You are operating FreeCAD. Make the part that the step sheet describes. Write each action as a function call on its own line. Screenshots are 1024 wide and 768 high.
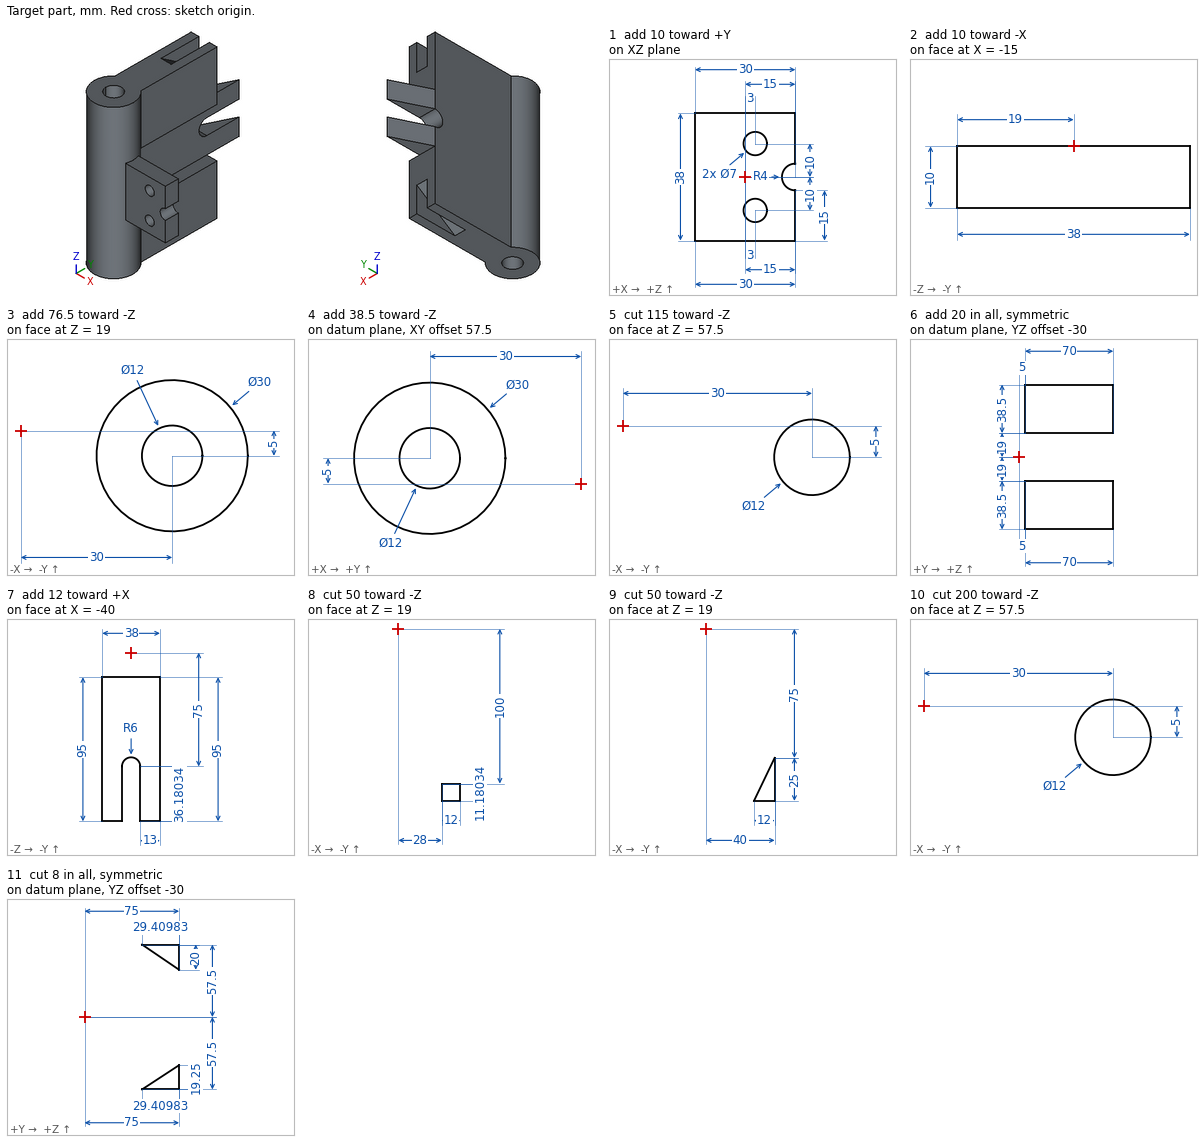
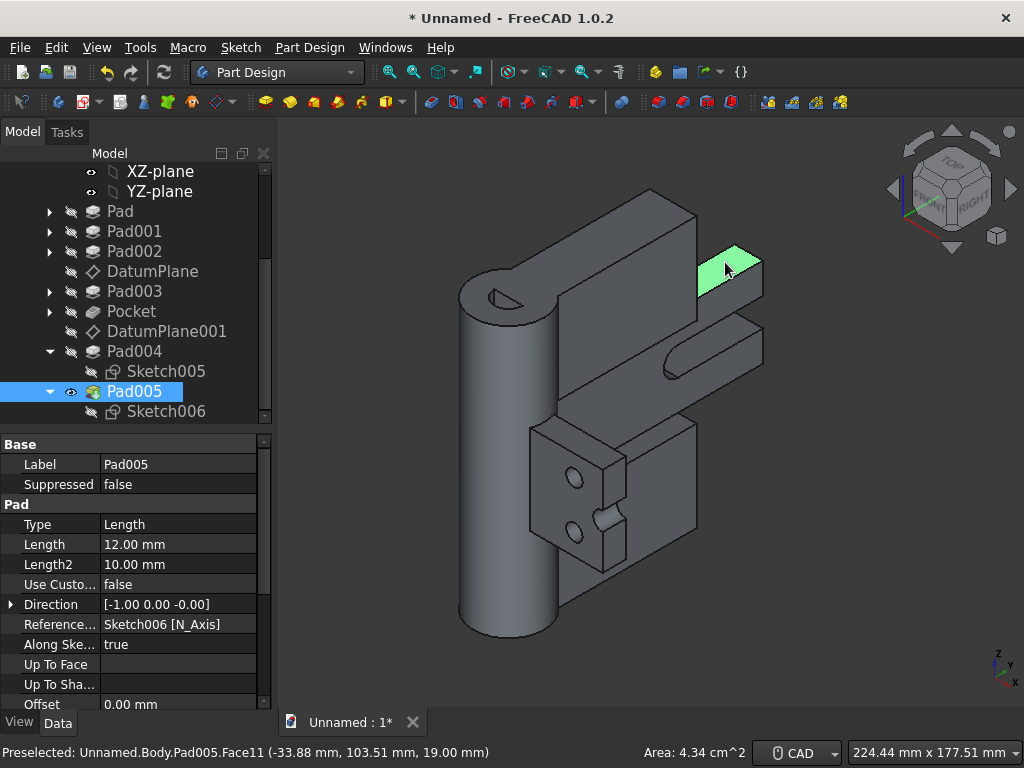
click(84, 102)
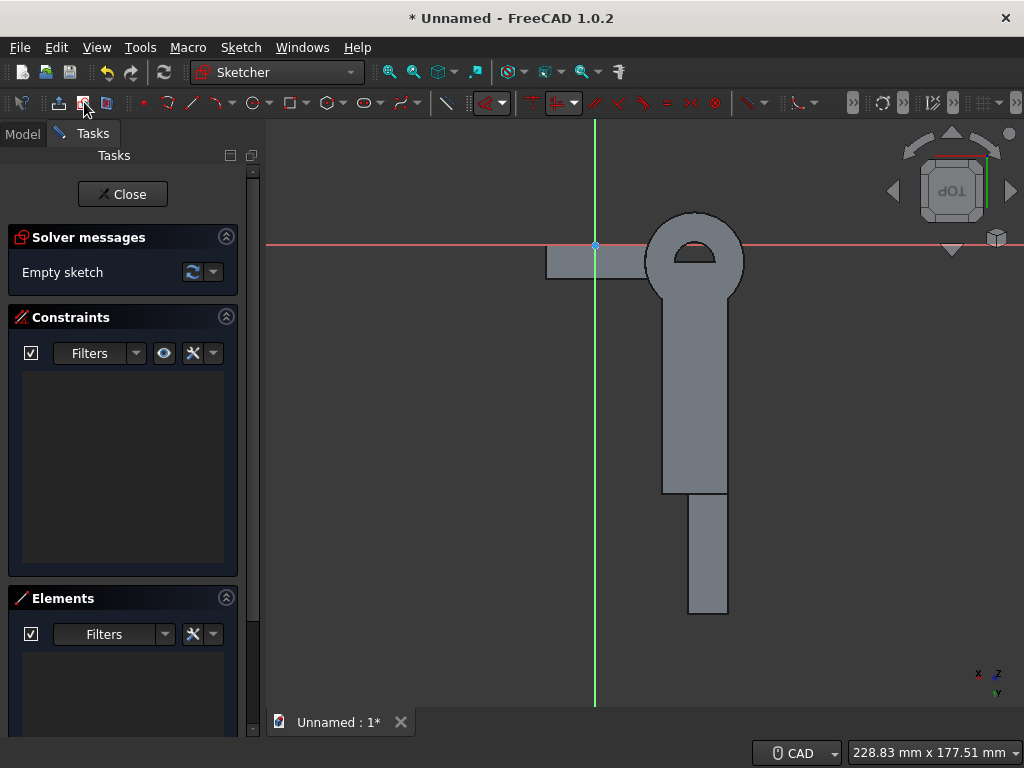
click(108, 104)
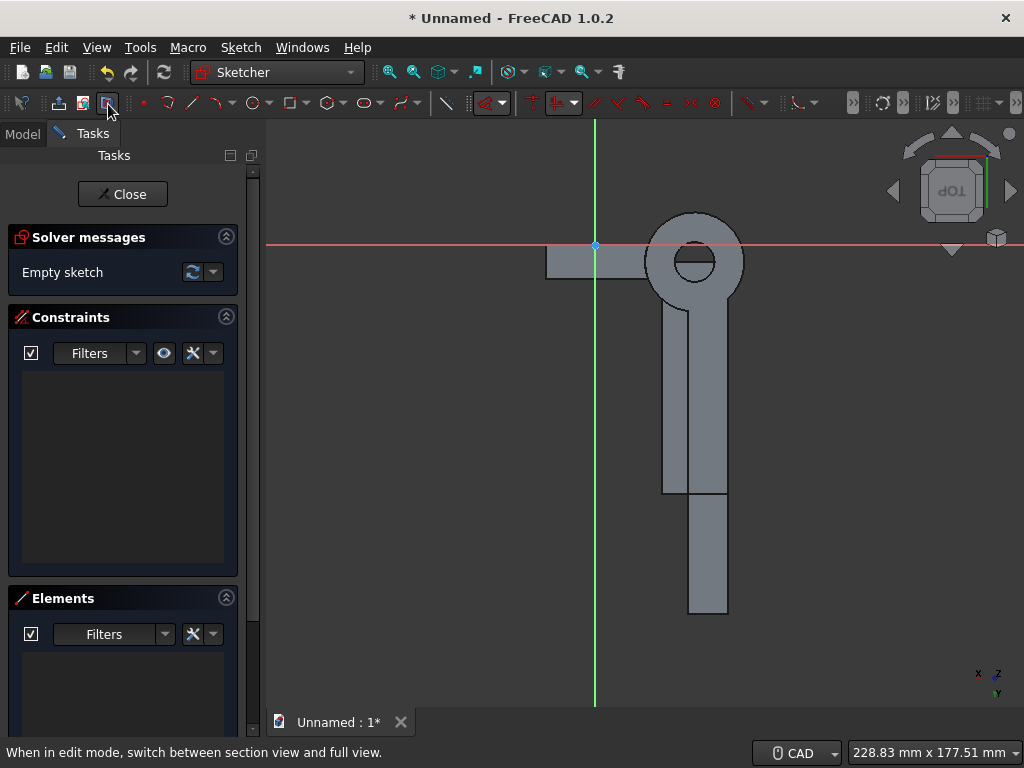
scroll(721, 613, up, 12)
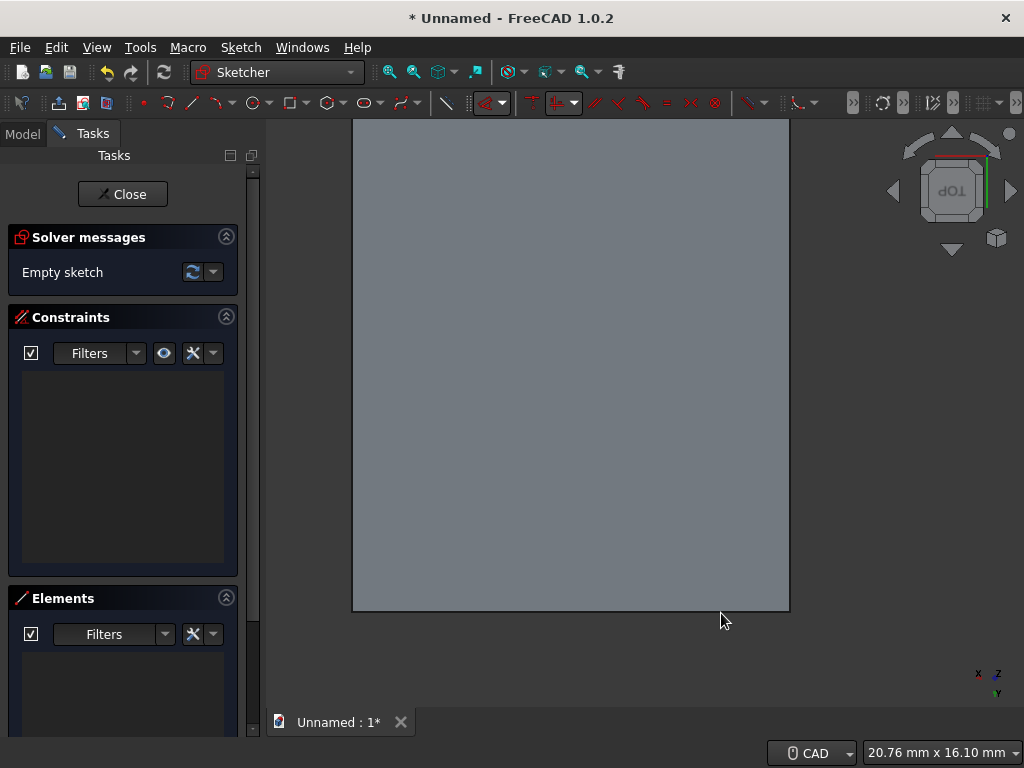
click(290, 104)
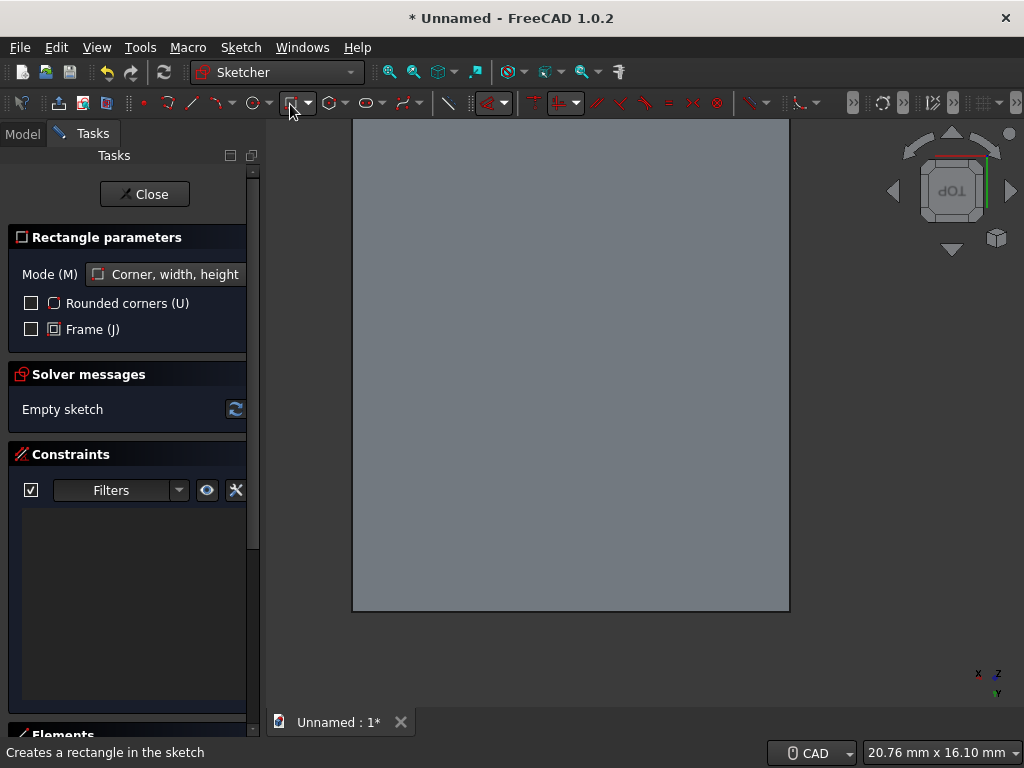
click(352, 204)
click(790, 612)
key(Escape)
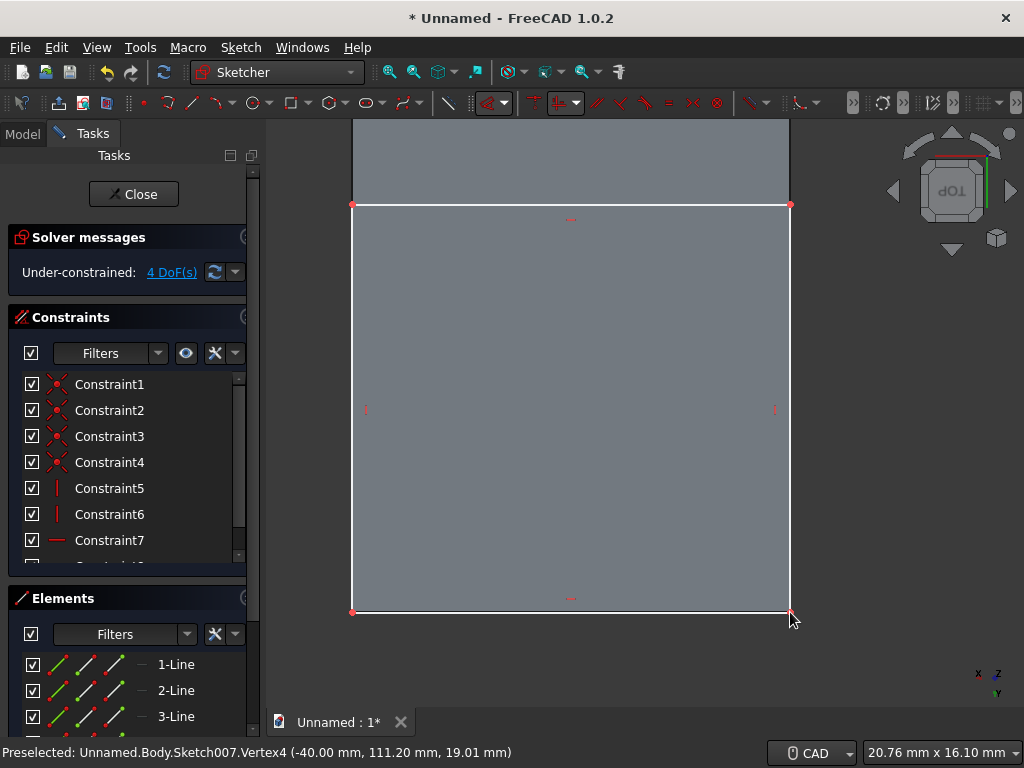
click(483, 613)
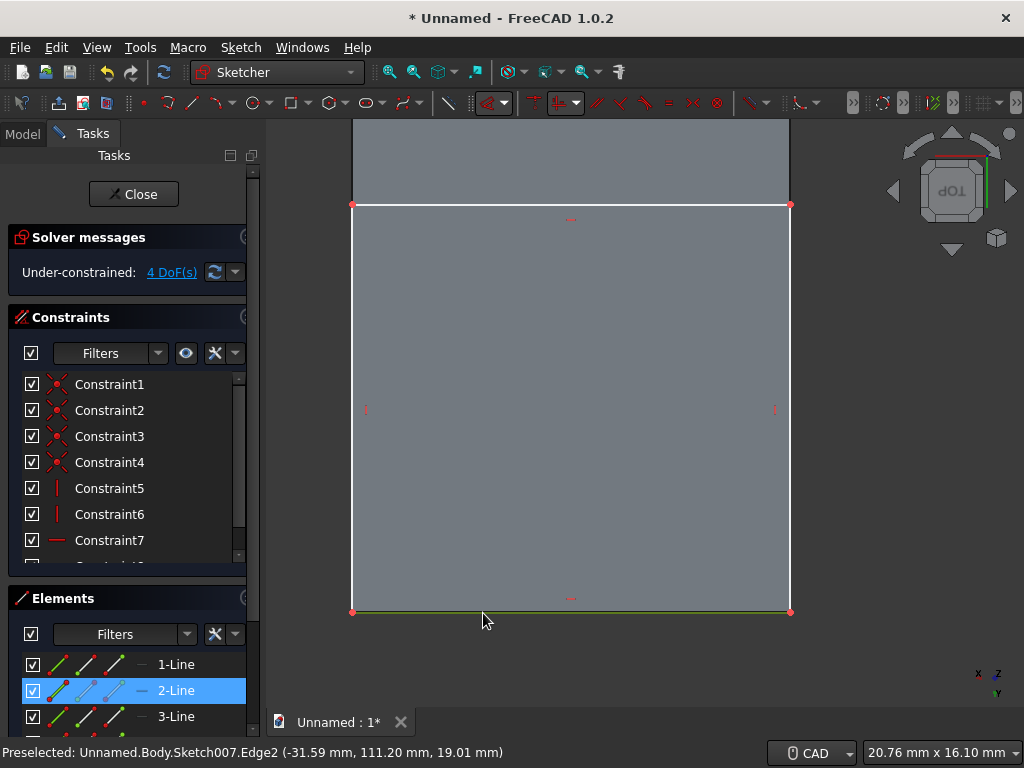
key(l)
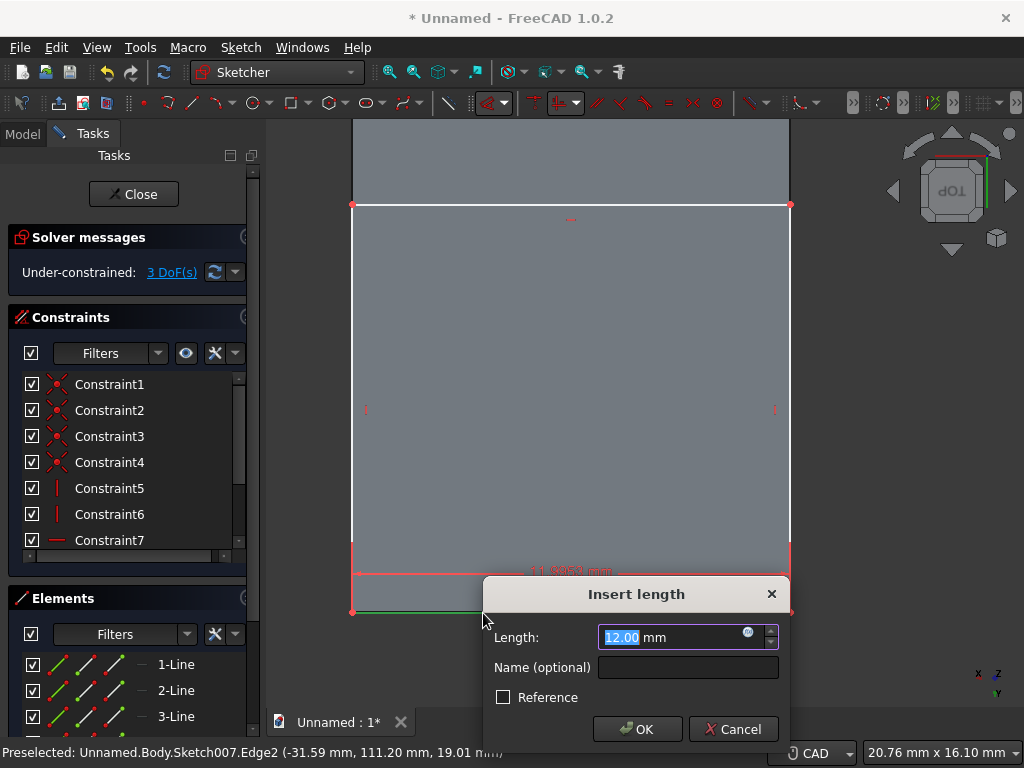
text(12)
key(Return)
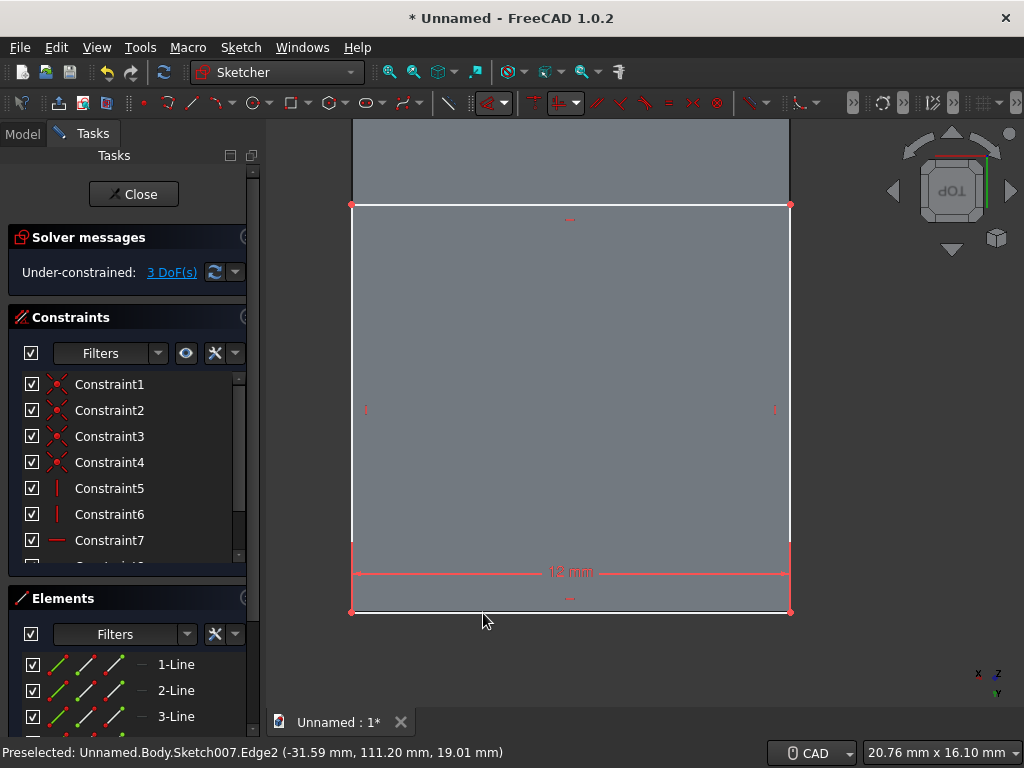
click(352, 205)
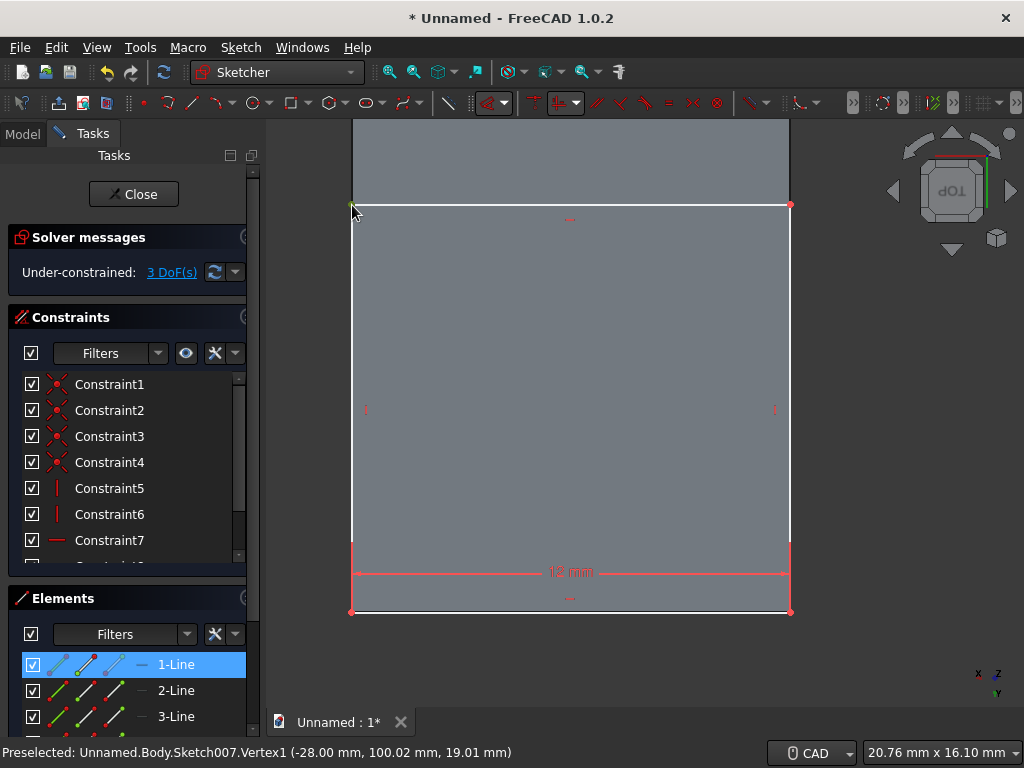
key(l)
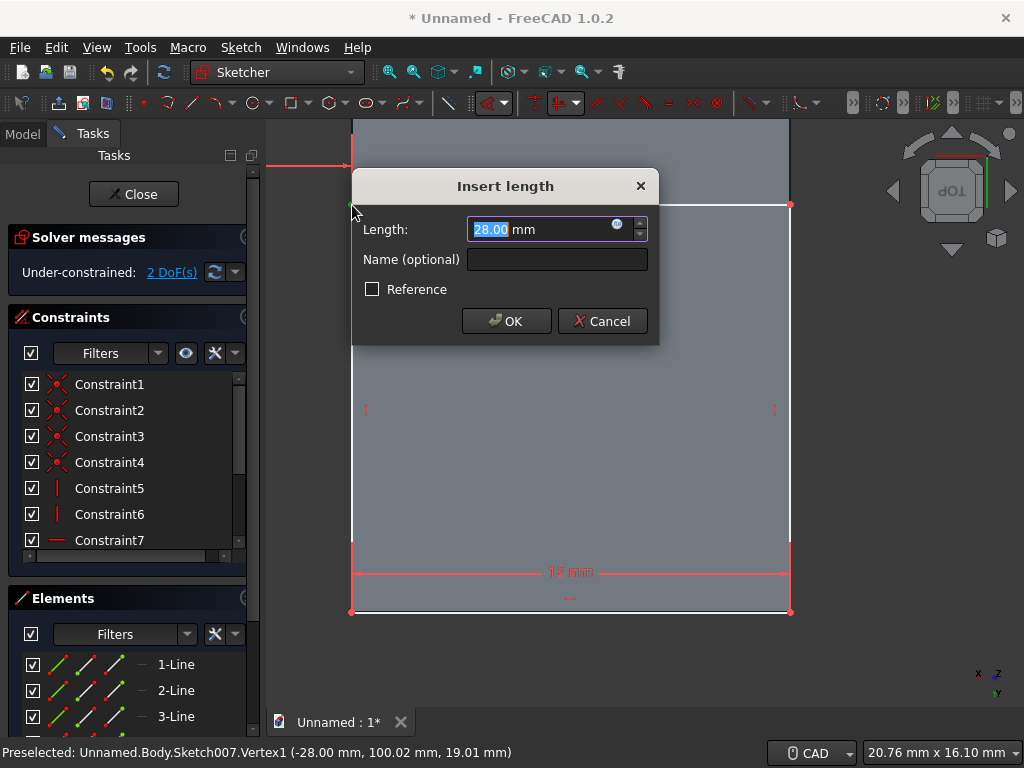
text(28)
key(Return)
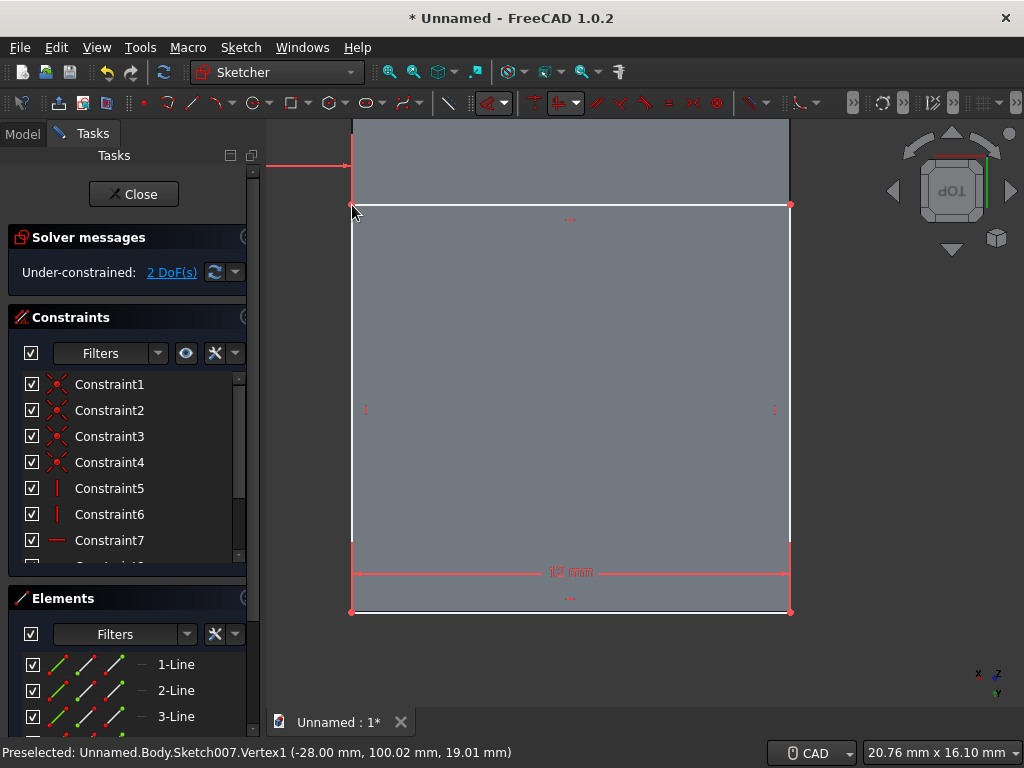
click(352, 205)